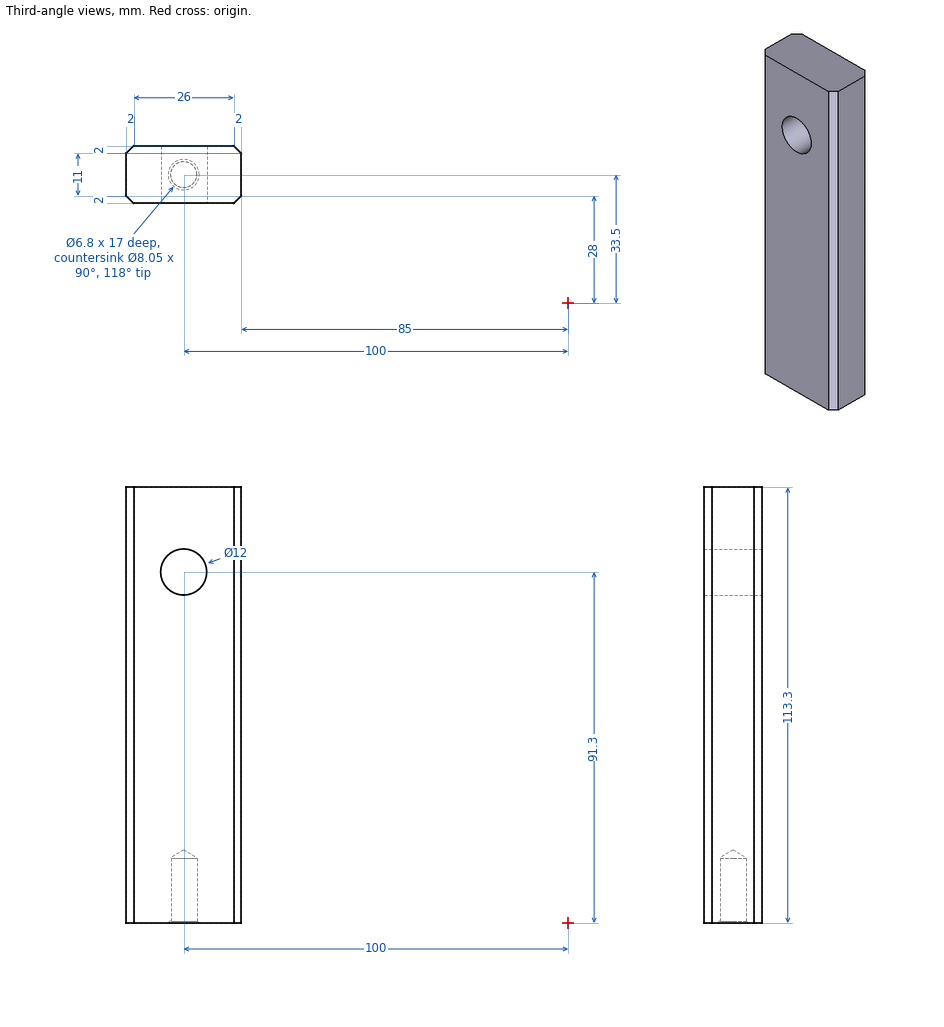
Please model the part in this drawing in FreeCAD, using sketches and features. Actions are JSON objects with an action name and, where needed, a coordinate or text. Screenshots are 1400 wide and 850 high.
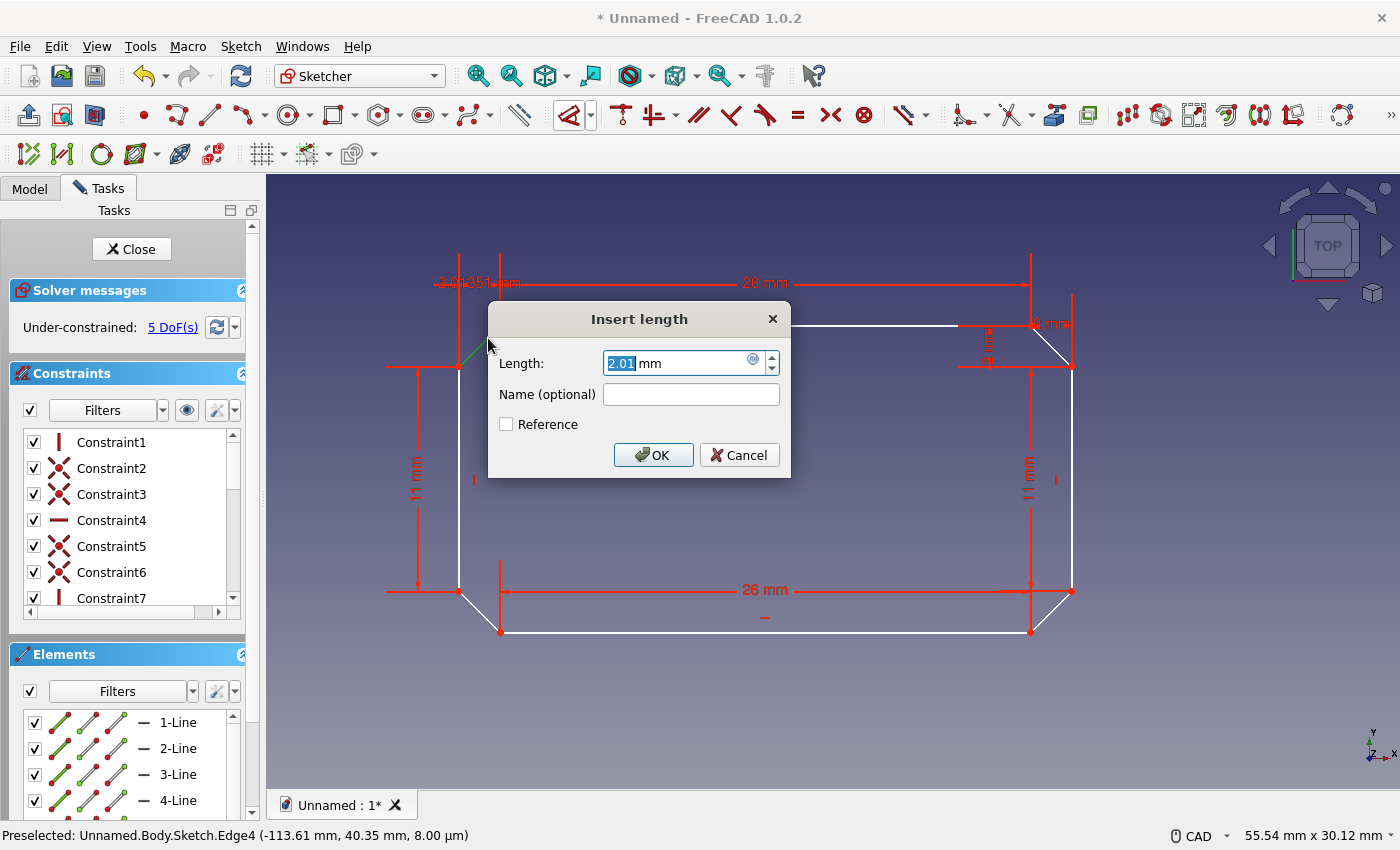
{"action": "type", "text": "2"}
{"action": "key", "text": "Return"}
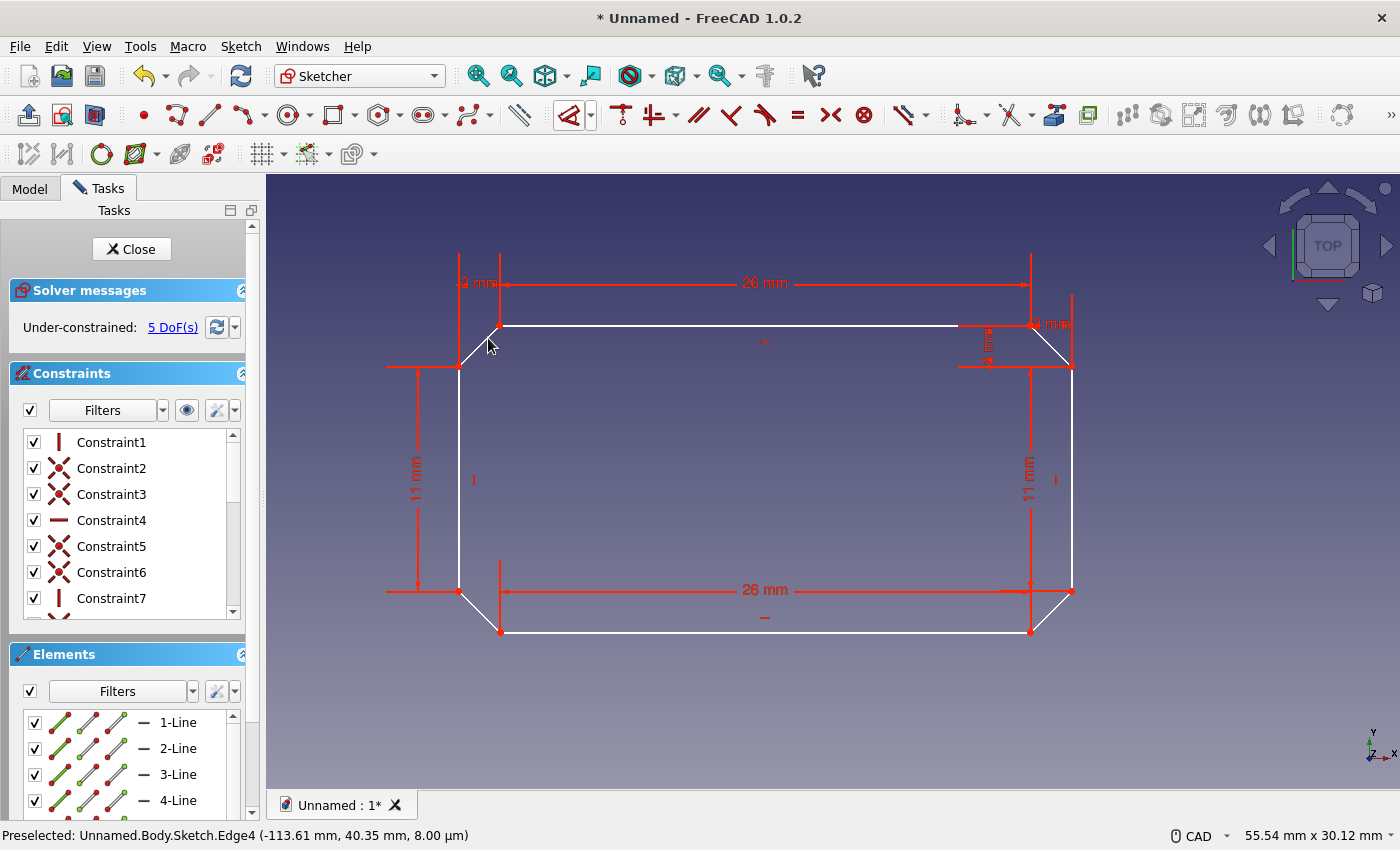
{"action": "left_click", "coordinate": [488, 338]}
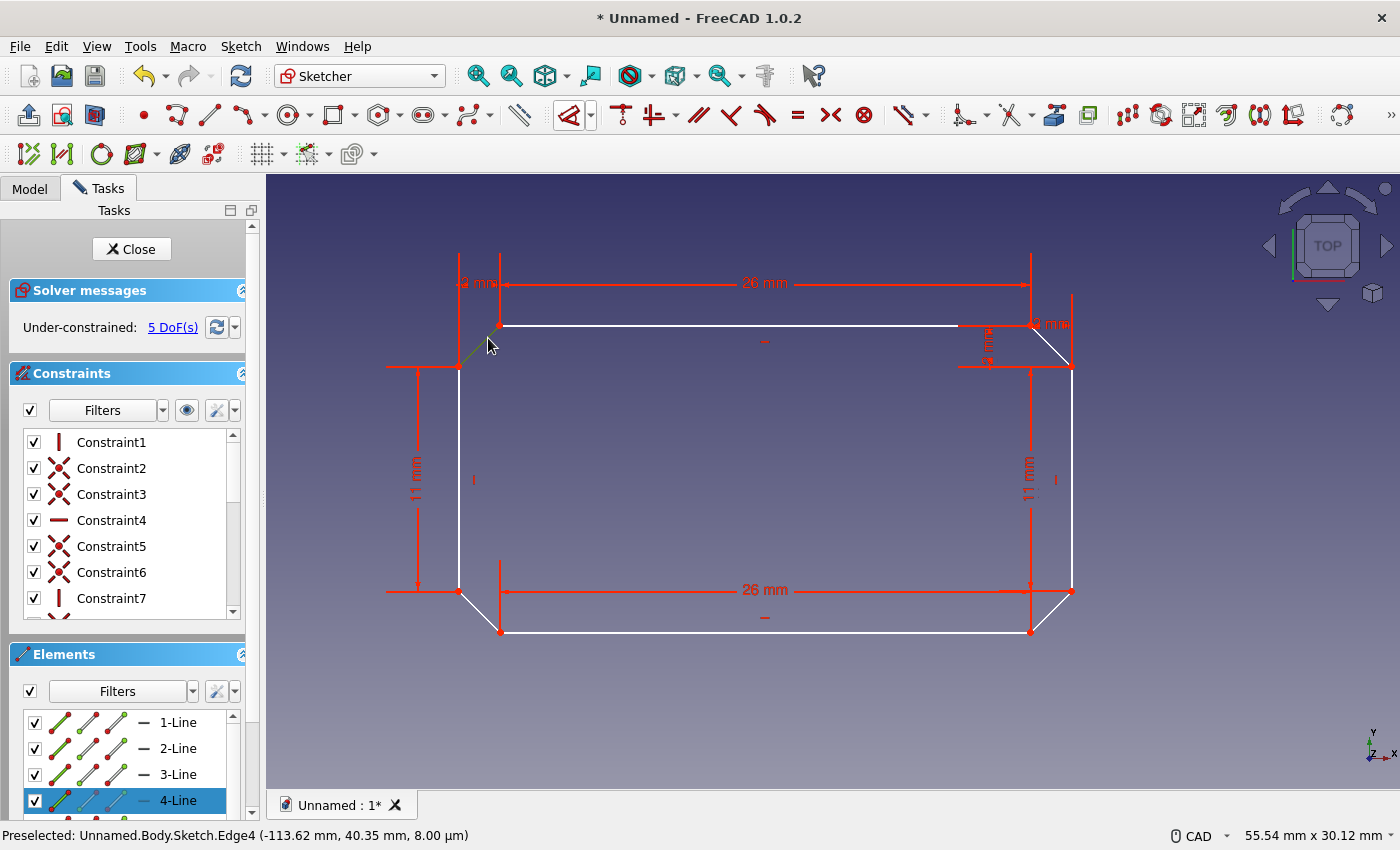
{"action": "left_click", "coordinate": [590, 116]}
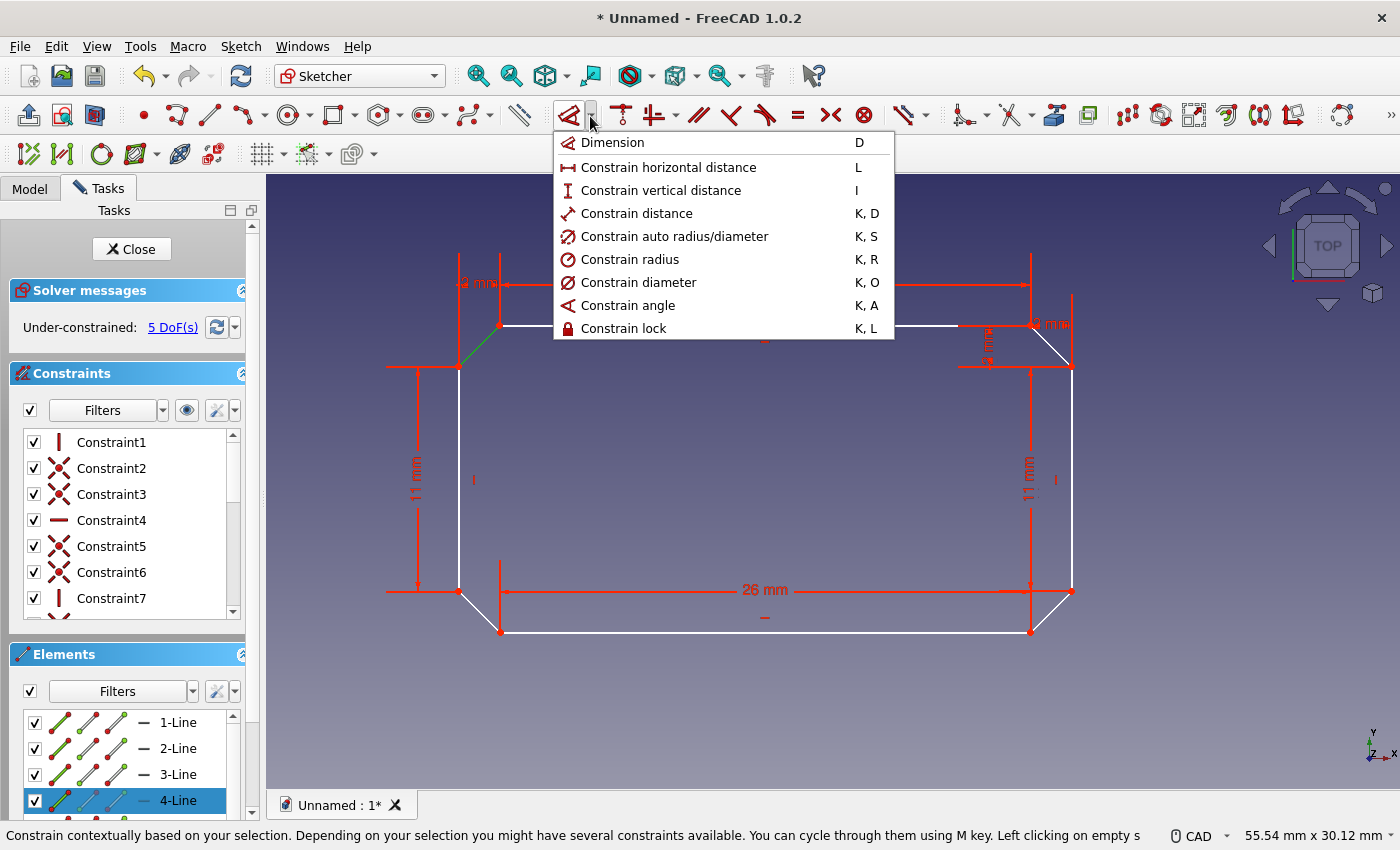
{"action": "left_click", "coordinate": [724, 190]}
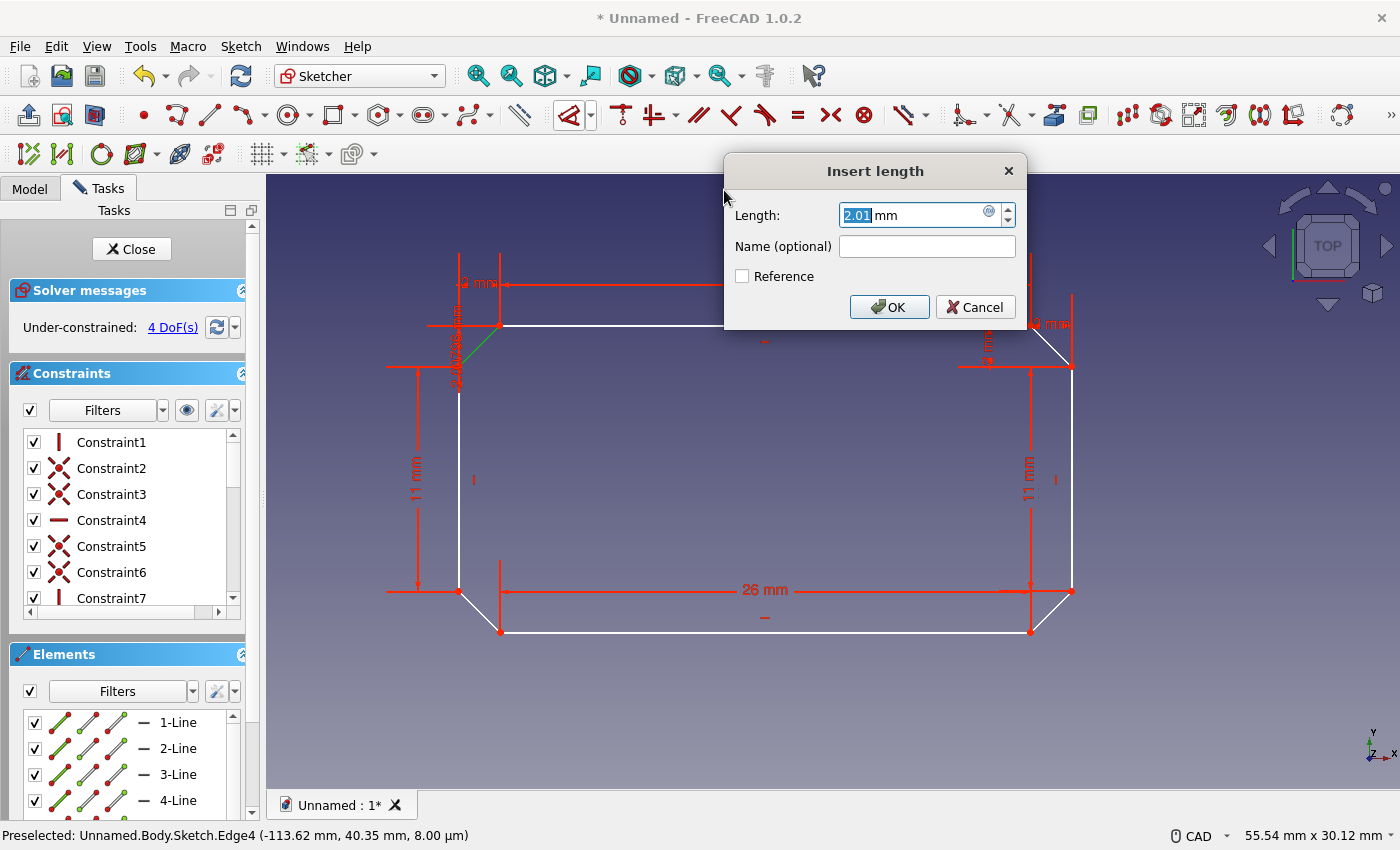
{"action": "type", "text": "2"}
{"action": "key", "text": "Return"}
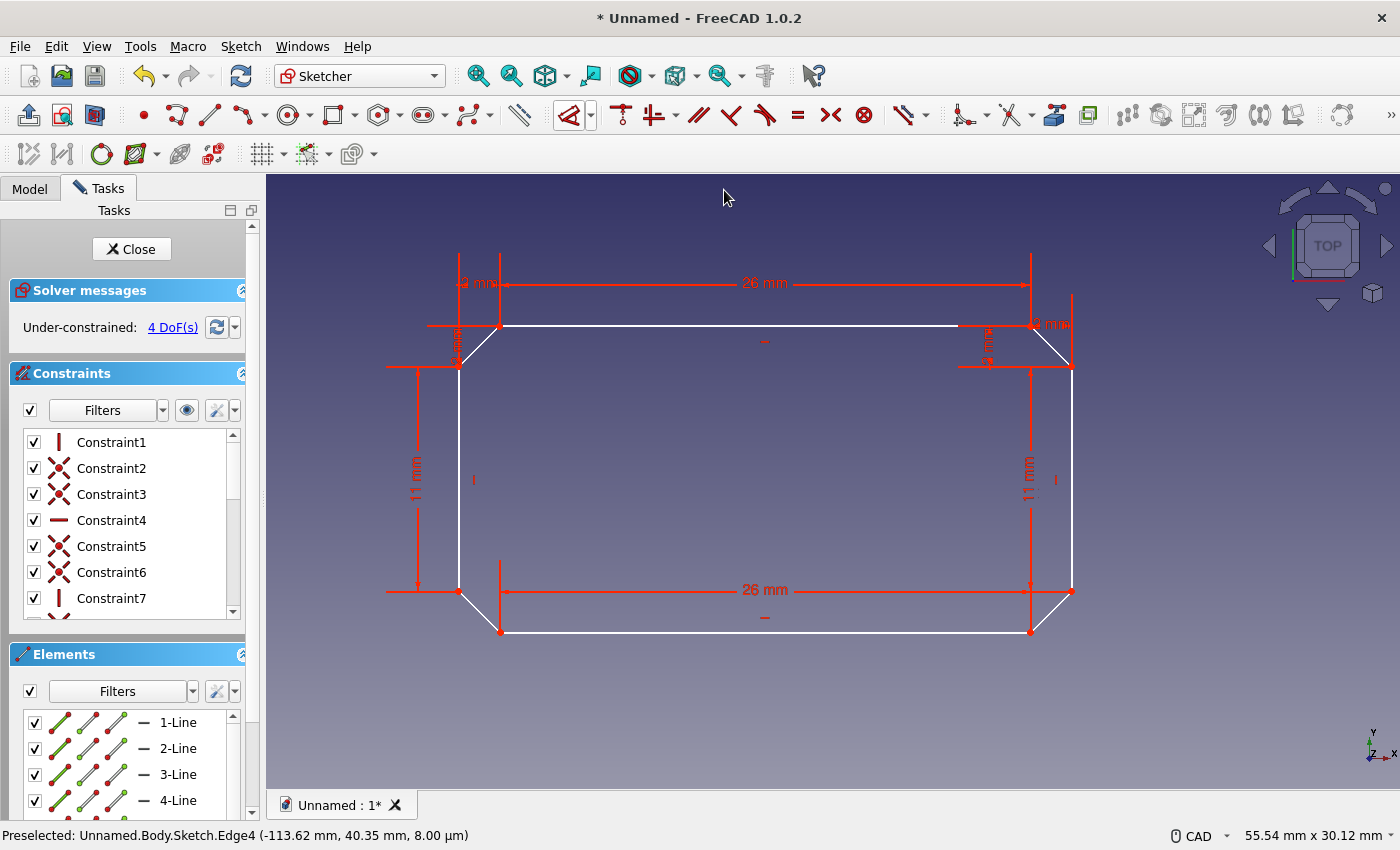
{"action": "left_click", "coordinate": [471, 604]}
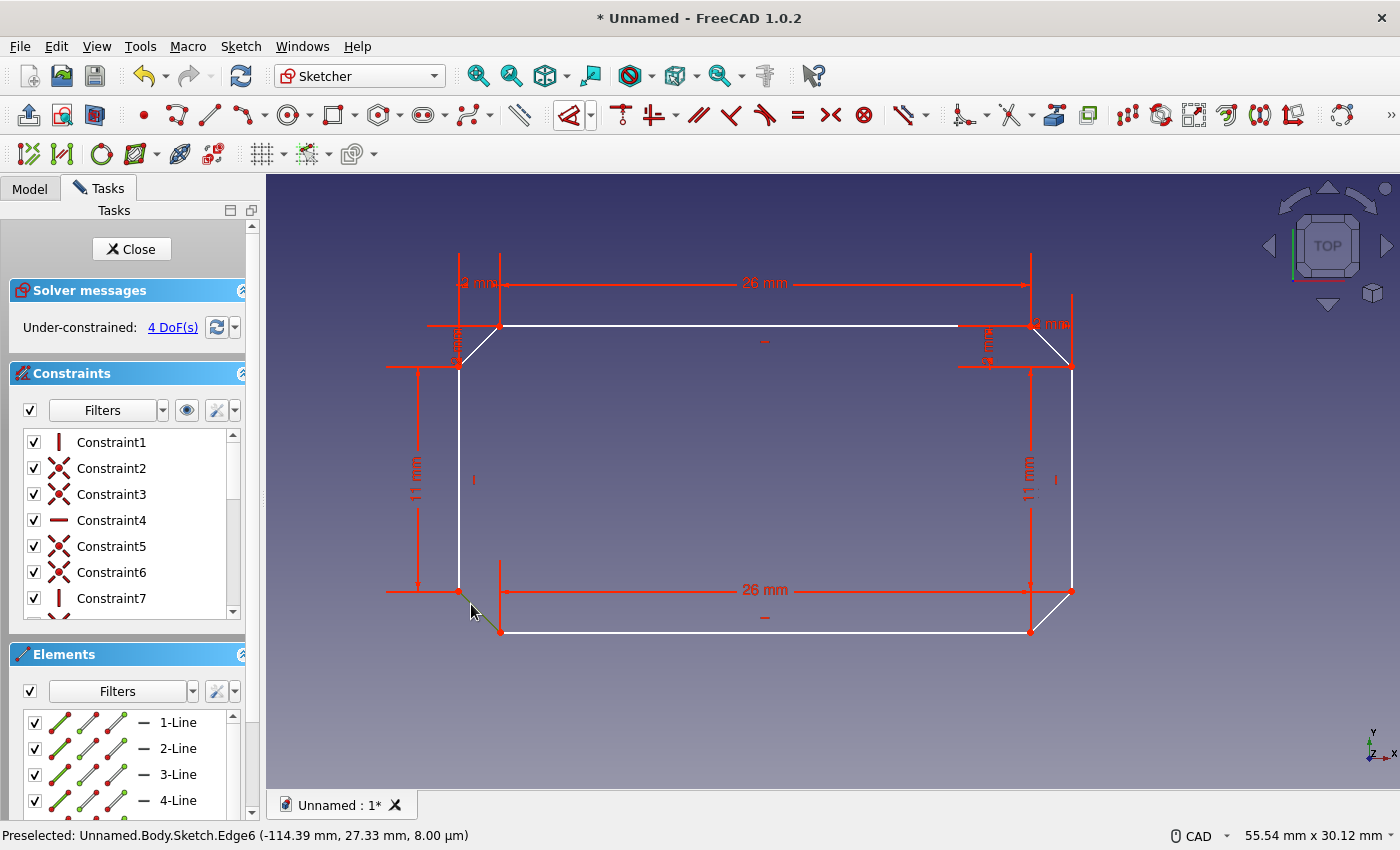
{"action": "key", "text": "l"}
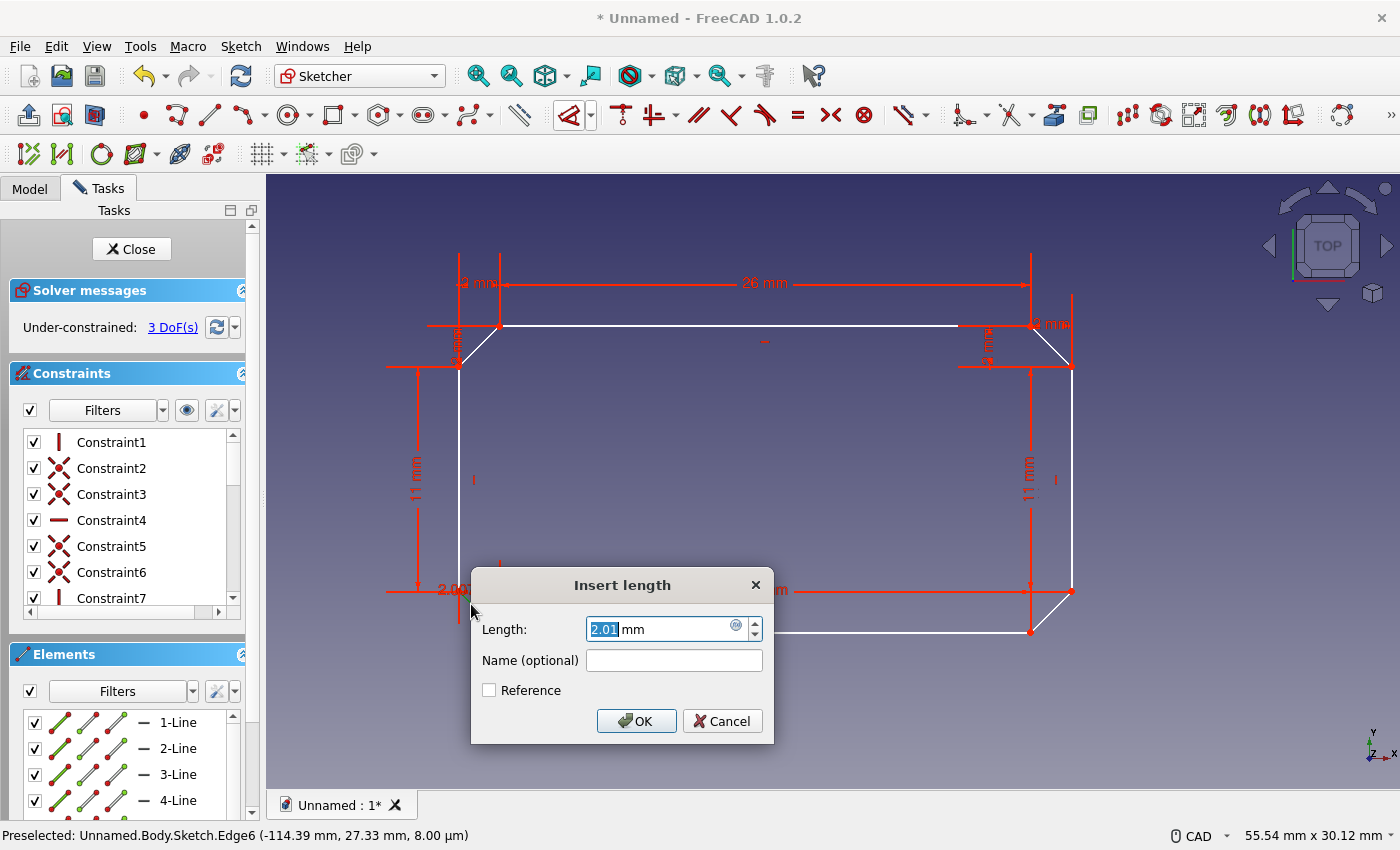
{"action": "type", "text": "2"}
{"action": "key", "text": "Return"}